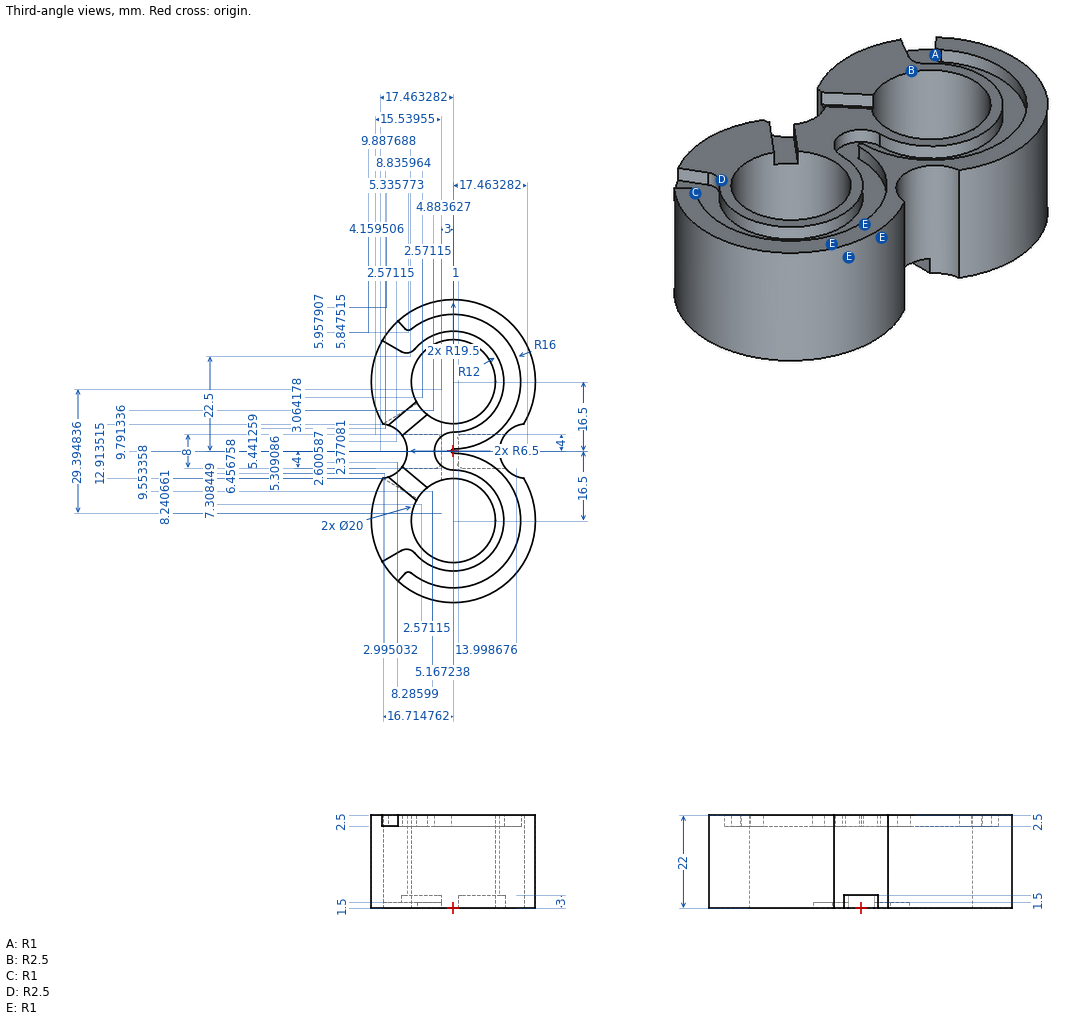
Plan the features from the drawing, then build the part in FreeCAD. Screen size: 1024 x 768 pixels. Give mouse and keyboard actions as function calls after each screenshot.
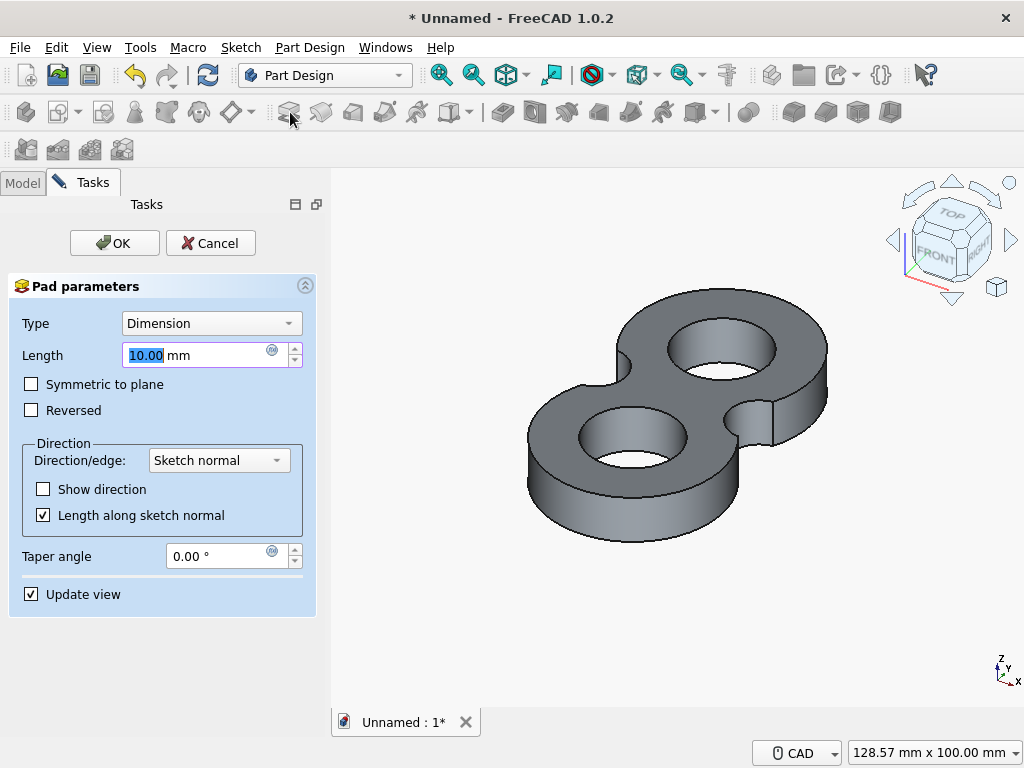
text(22)
key(Tab)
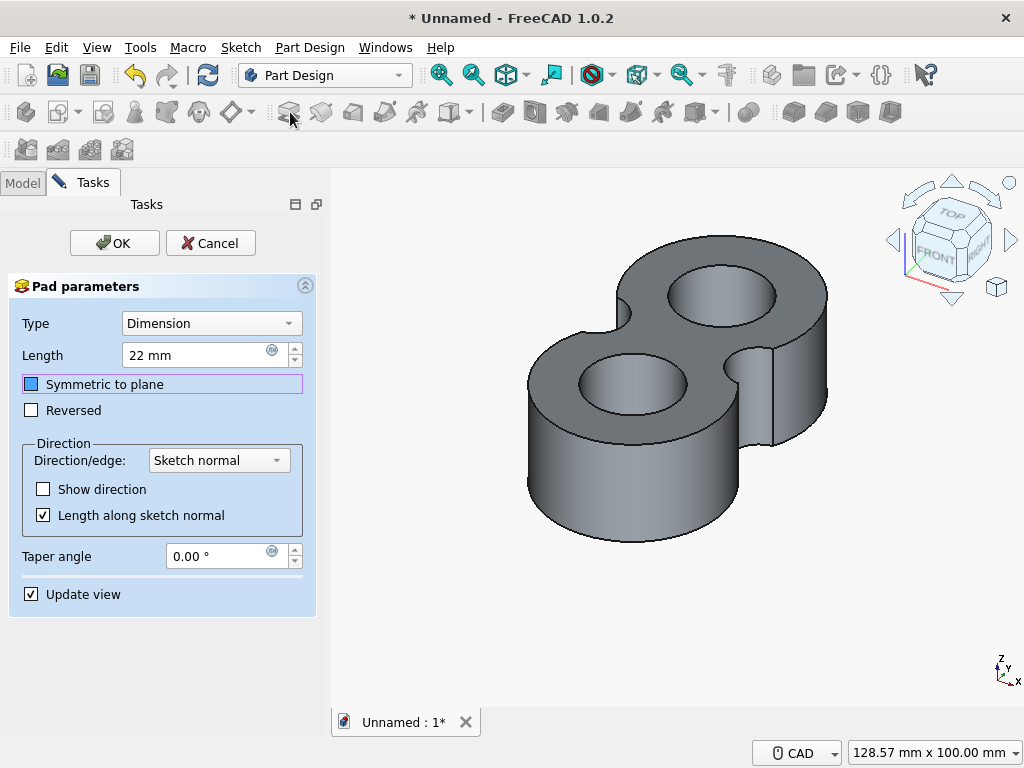
click(115, 243)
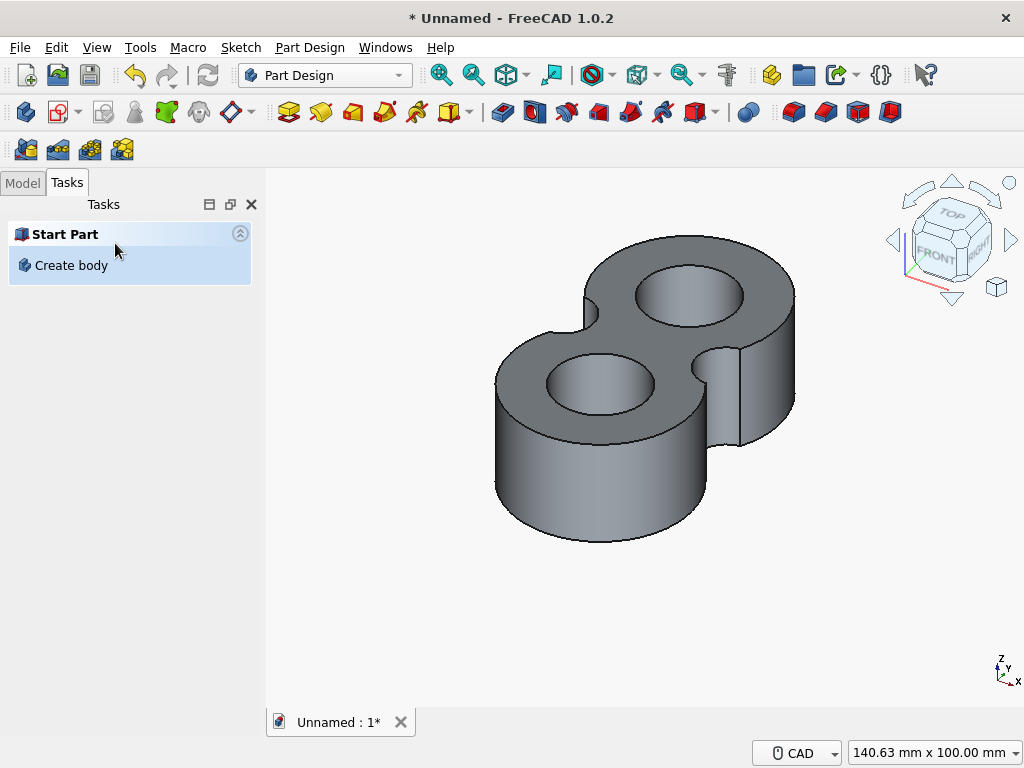
click(645, 339)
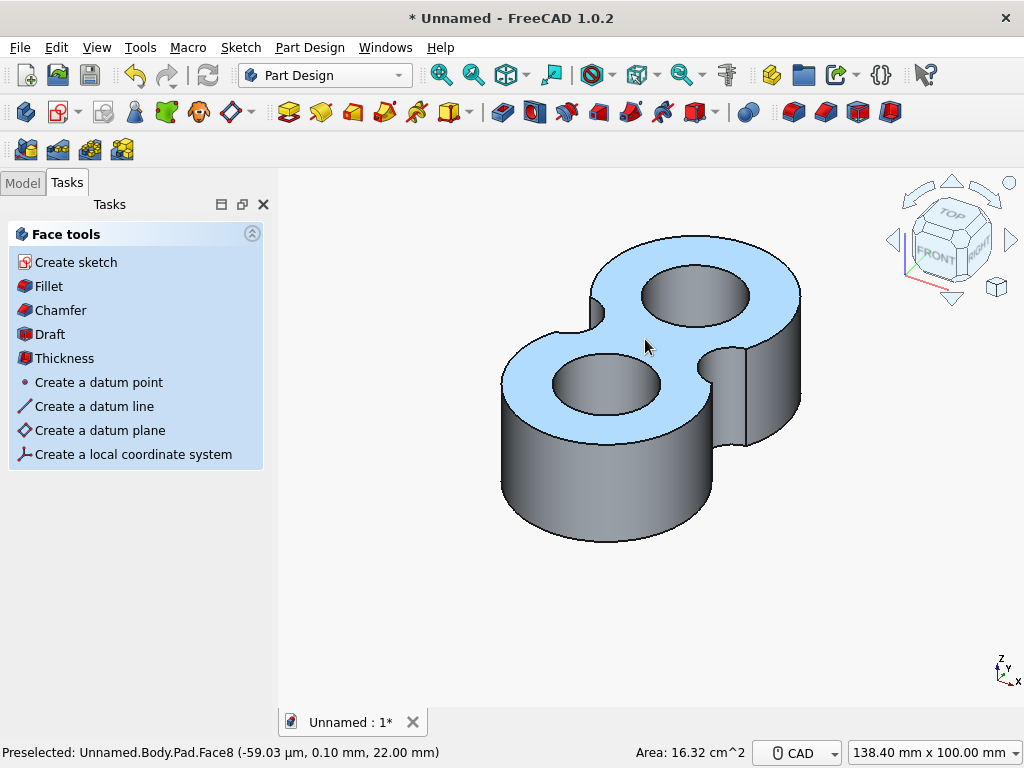
click(58, 112)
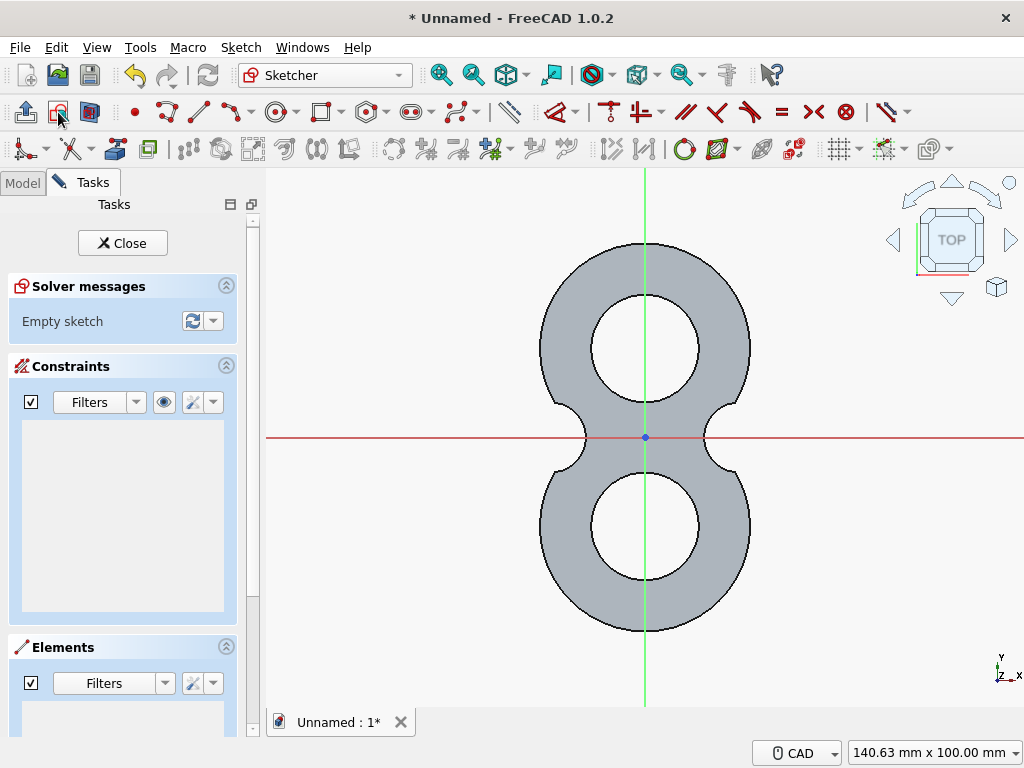
scroll(696, 233, up, 3)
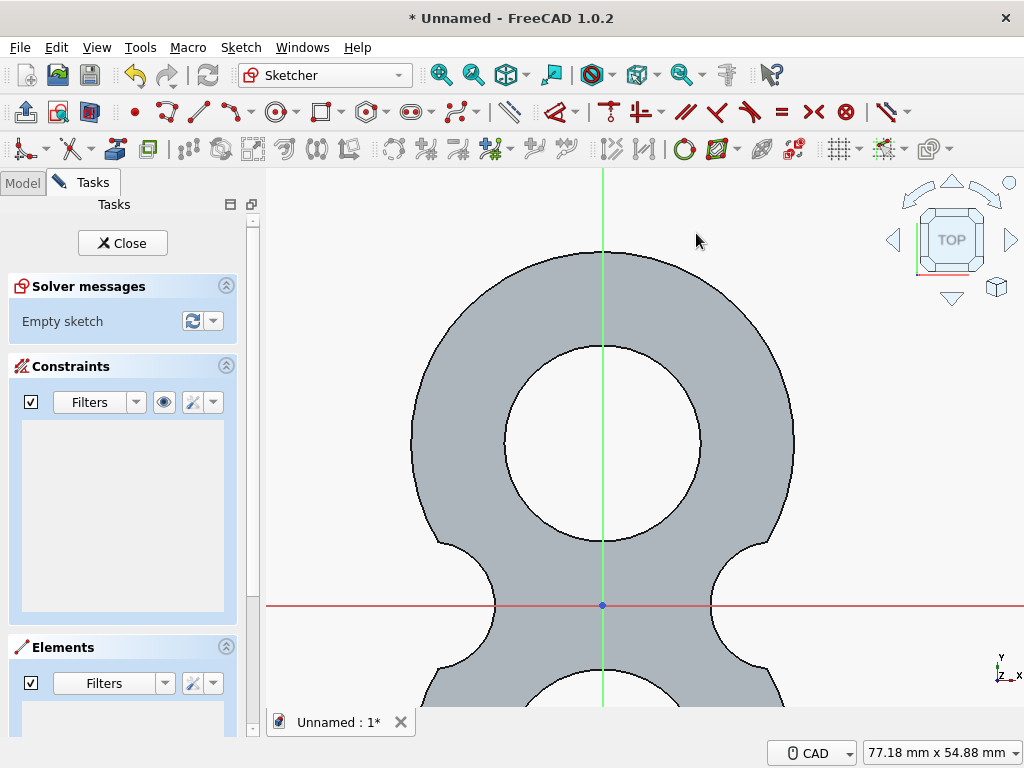
key(g)
key(l)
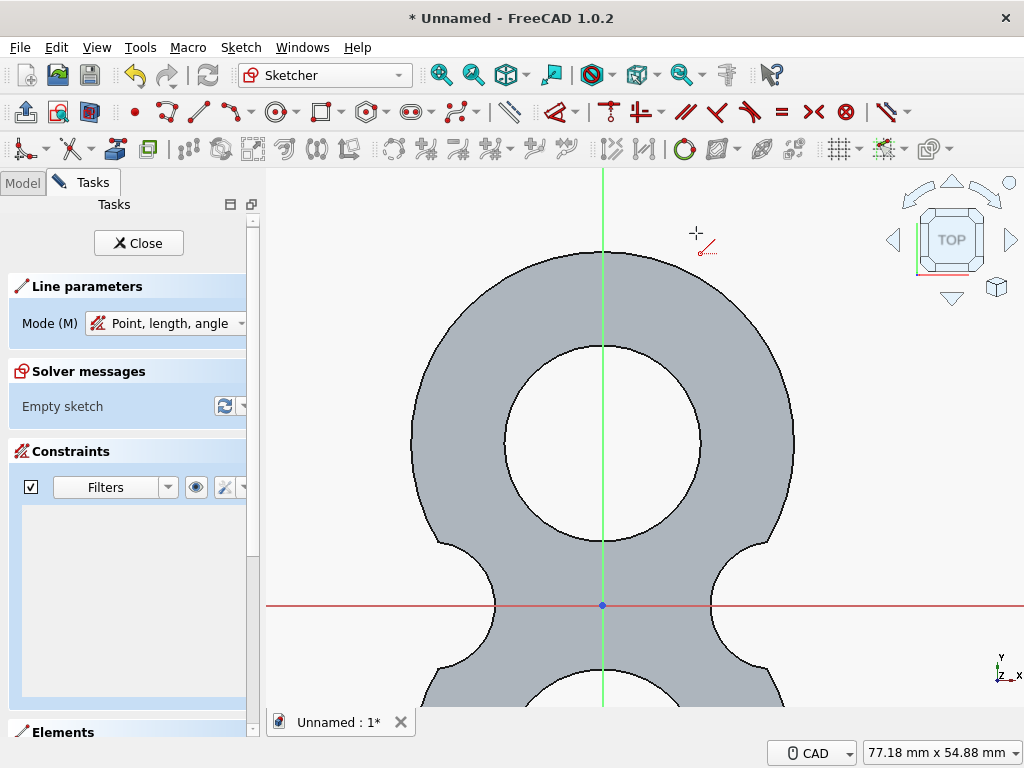
click(558, 606)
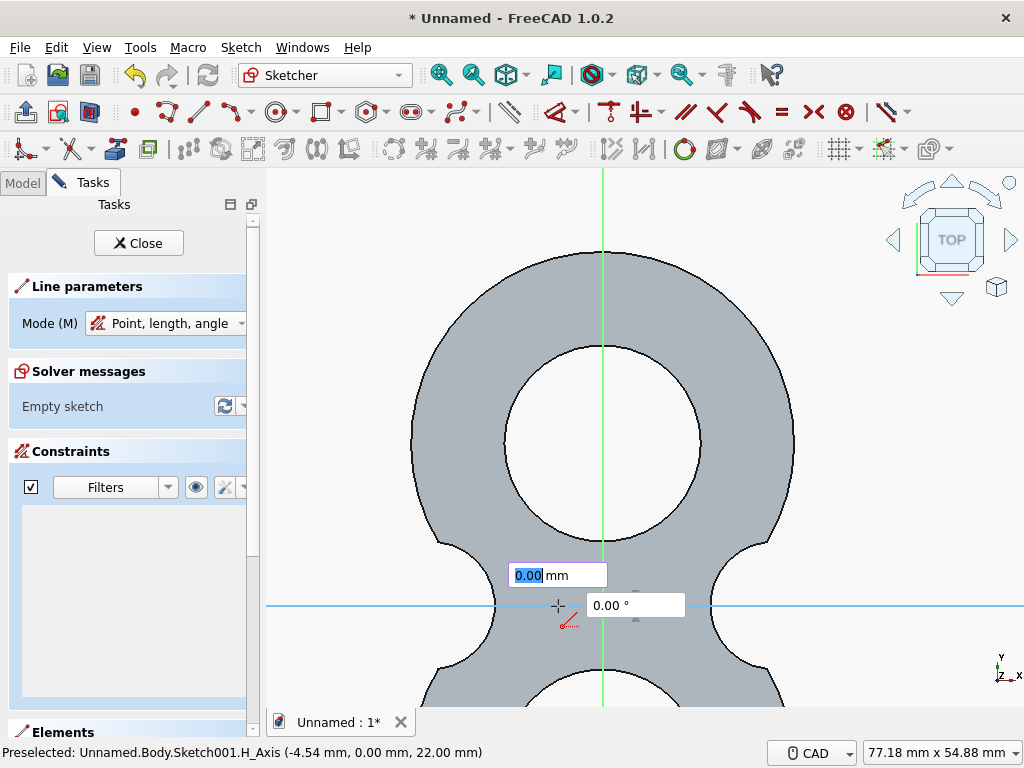
scroll(598, 606, up, 6)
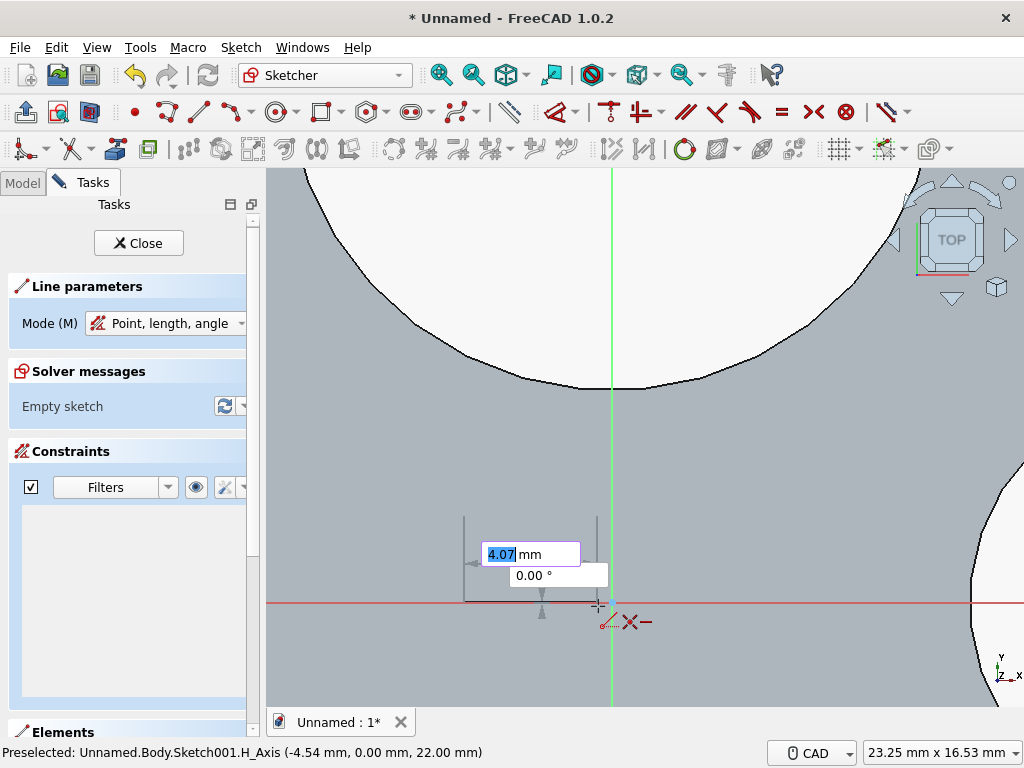
click(596, 594)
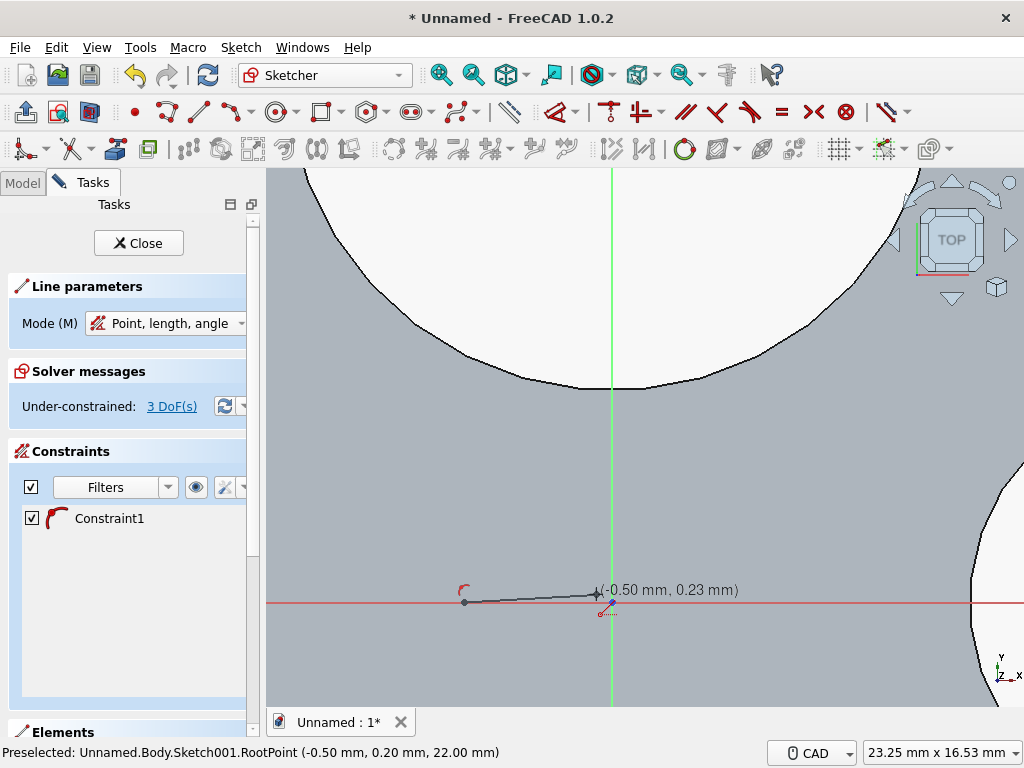
click(168, 112)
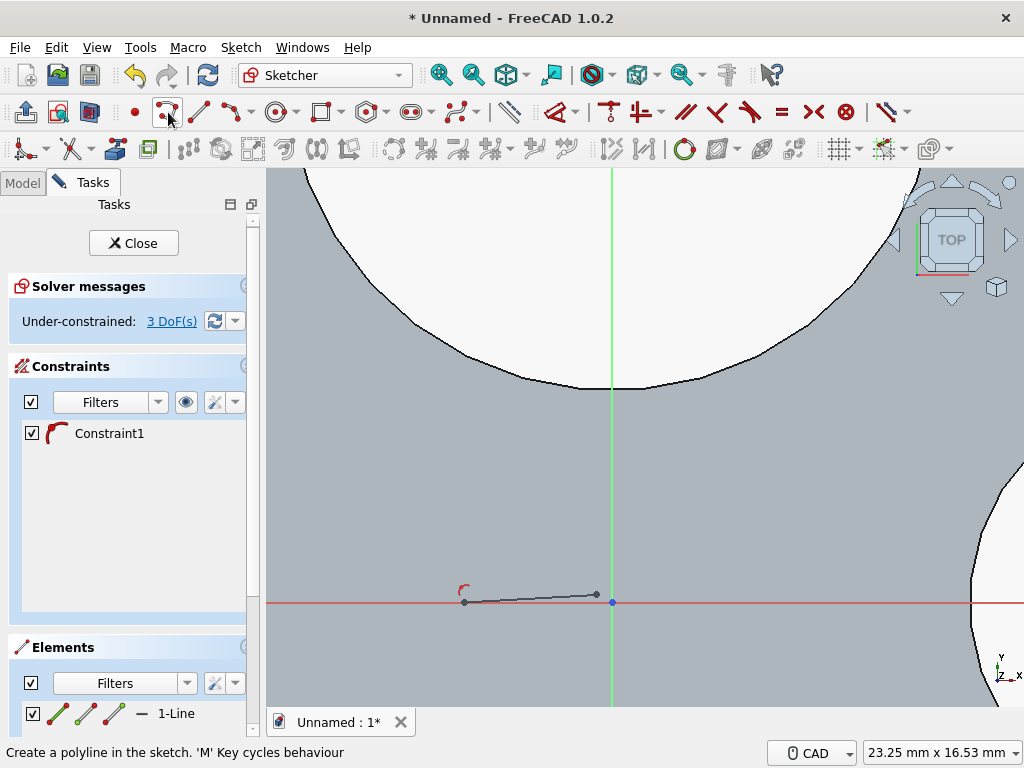
scroll(599, 606, down, 6)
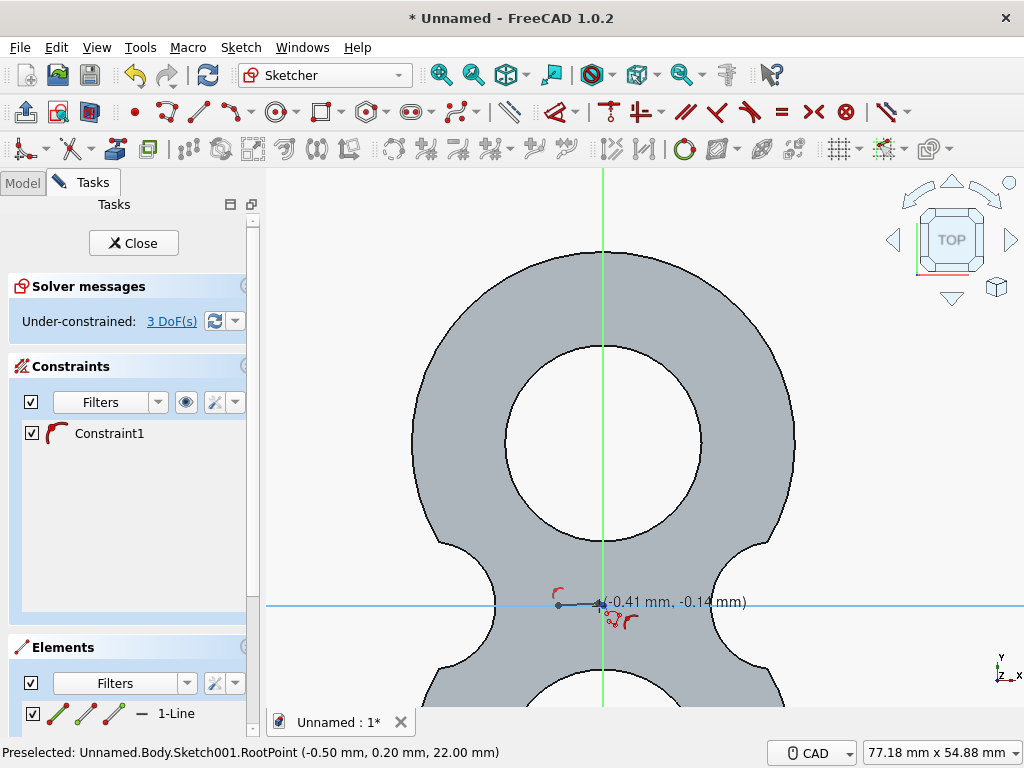
click(497, 327)
click(445, 270)
click(404, 328)
click(501, 385)
right_click(501, 385)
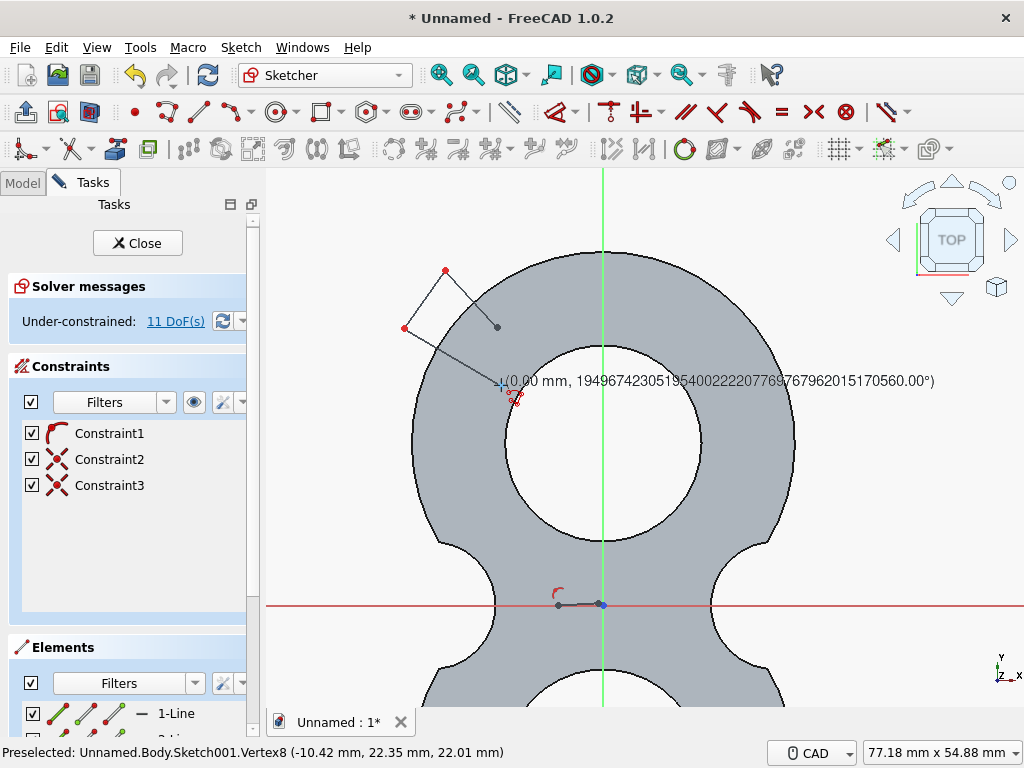
key(g)
key(3)
key(a)